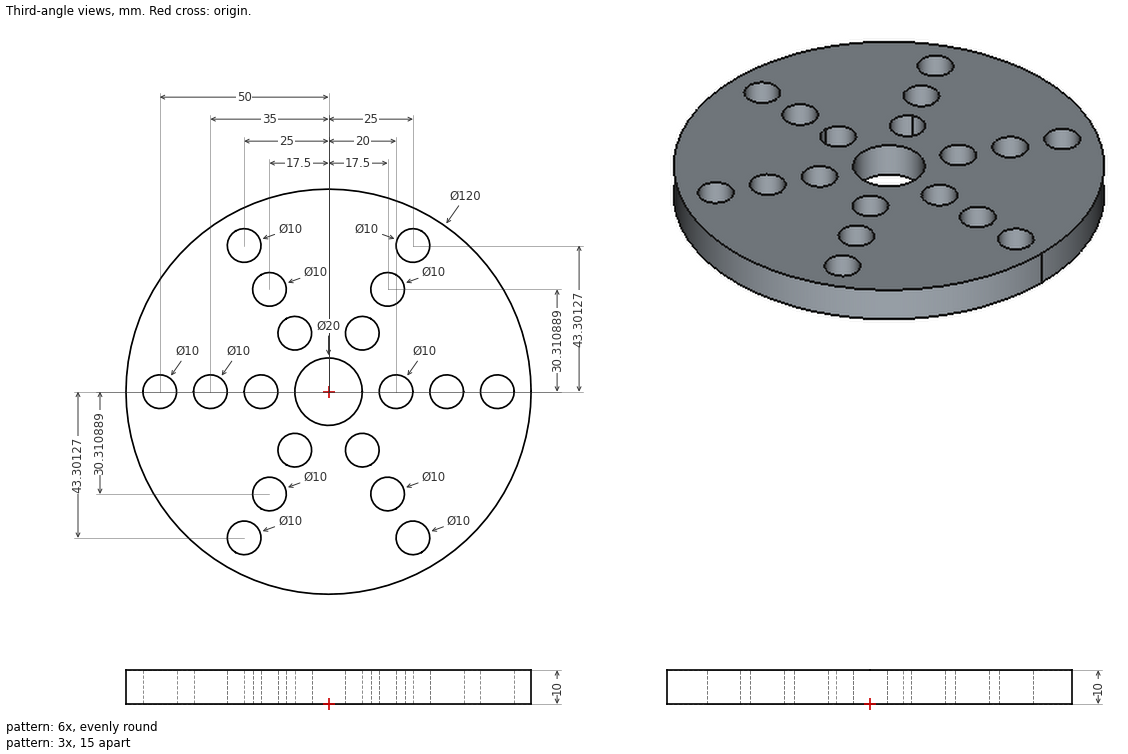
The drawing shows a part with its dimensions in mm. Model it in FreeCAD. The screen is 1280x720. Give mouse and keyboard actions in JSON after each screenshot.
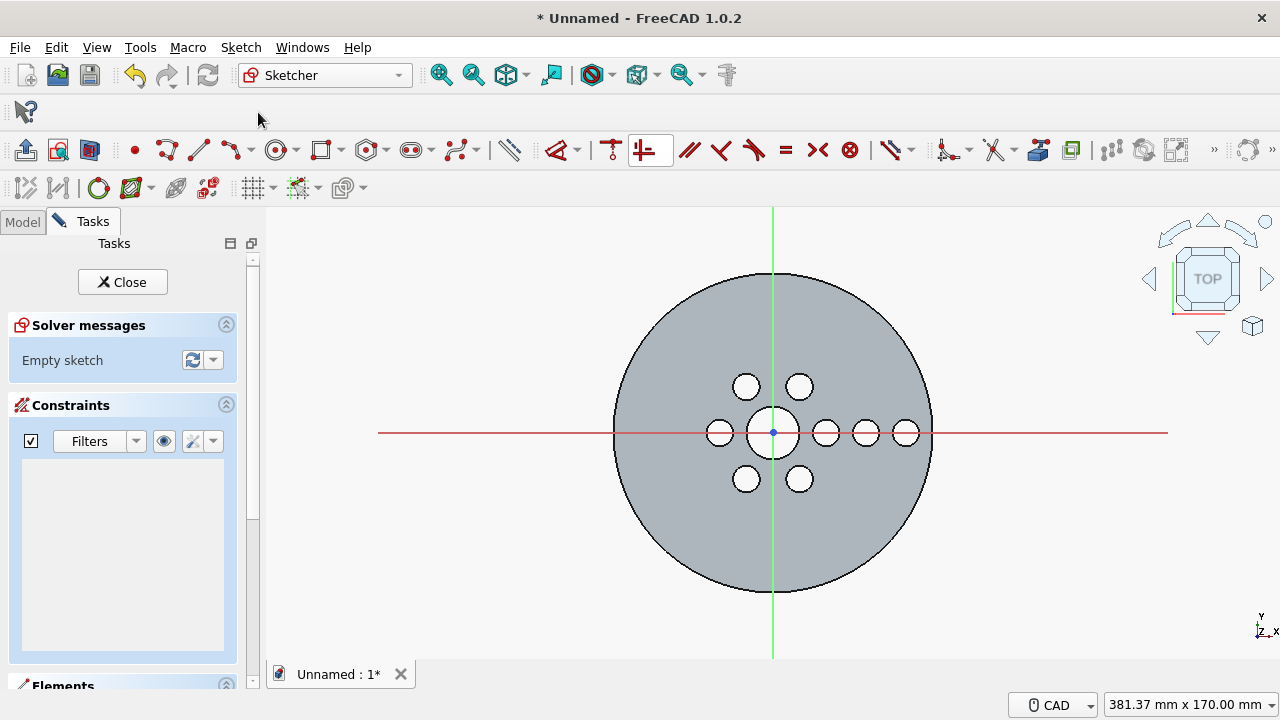
{"action": "scroll", "coordinate": [831, 344], "scroll_direction": "up", "scroll_amount": 12}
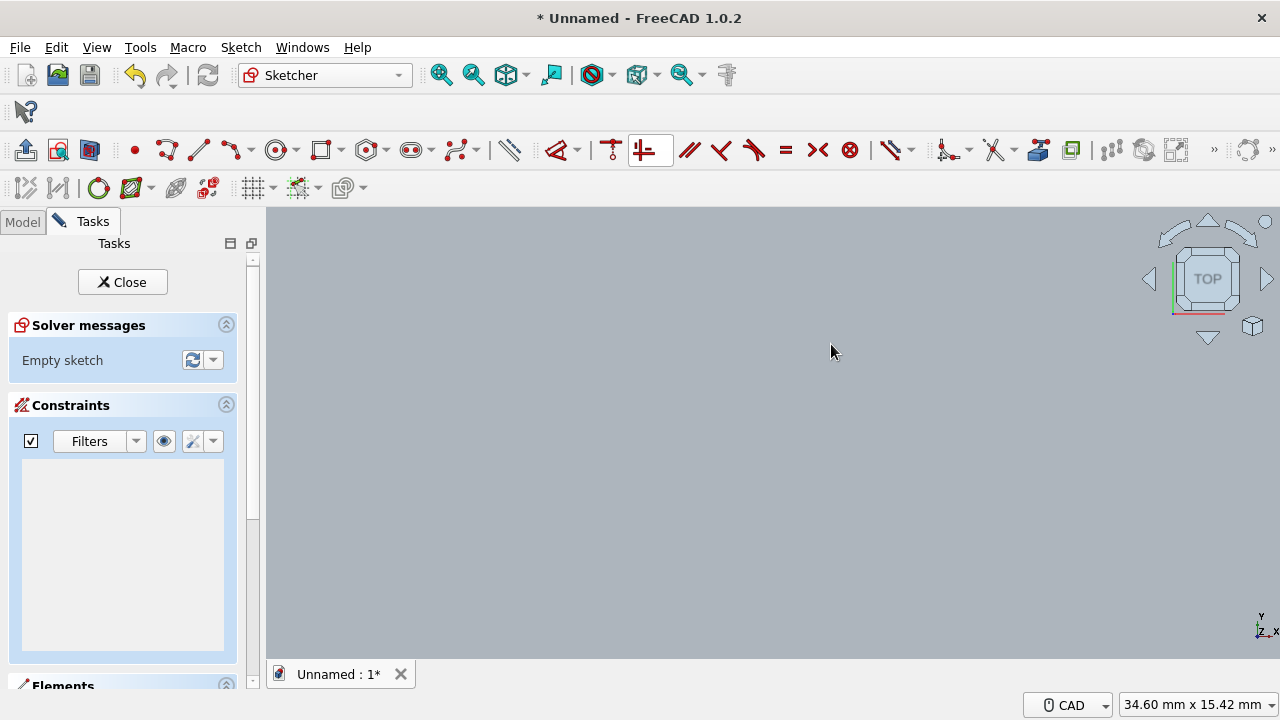
{"action": "left_click", "coordinate": [276, 150]}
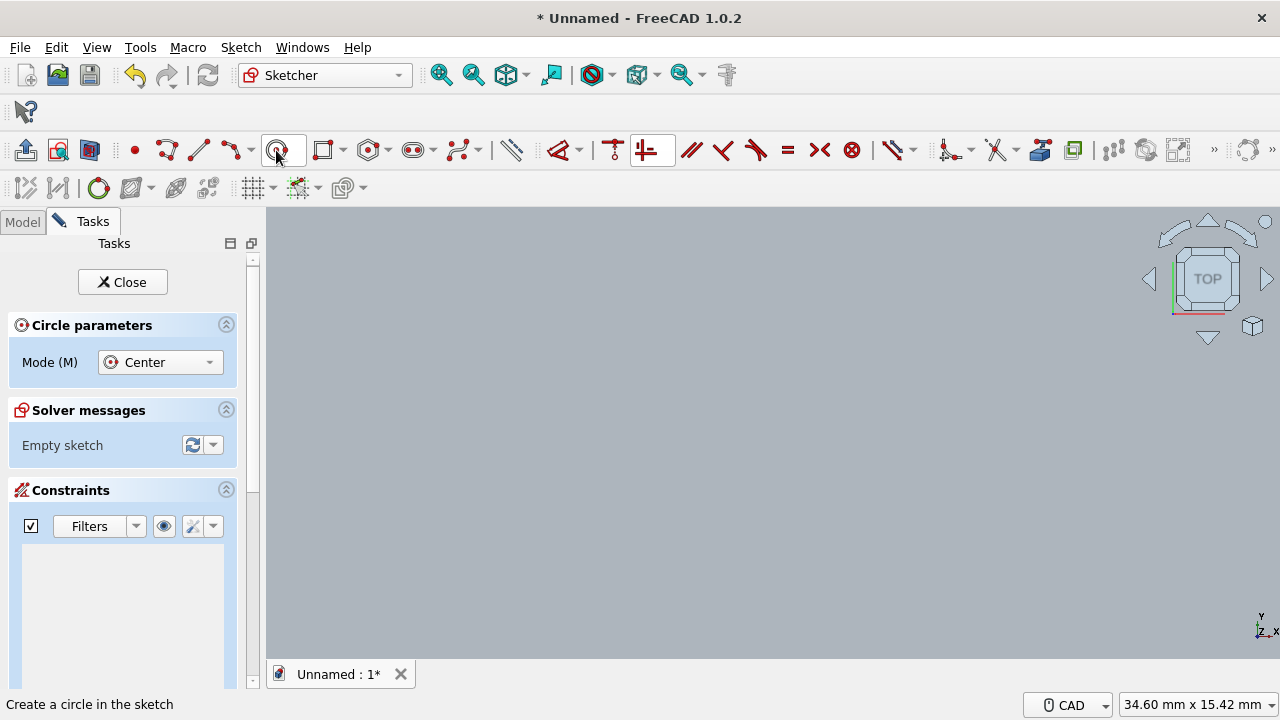
{"action": "left_click", "coordinate": [699, 434]}
{"action": "left_click", "coordinate": [803, 330]}
{"action": "key", "text": "Escape"}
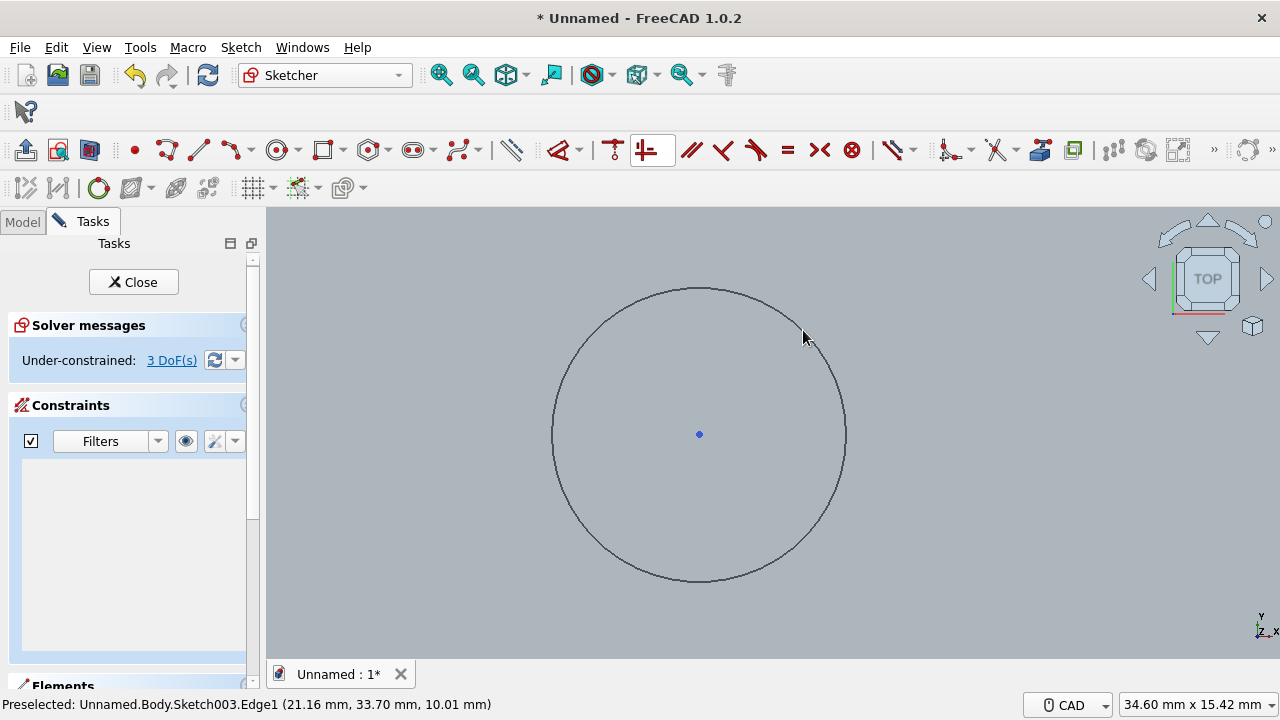
{"action": "left_click", "coordinate": [558, 150]}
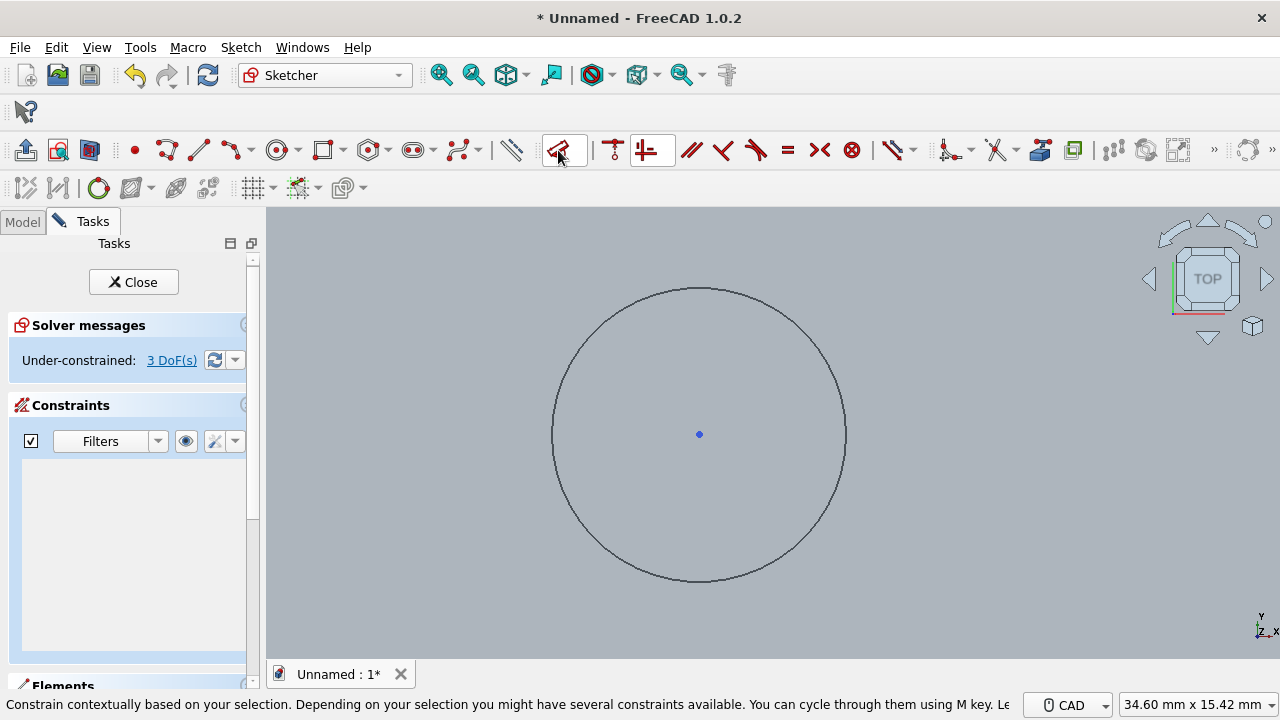
{"action": "left_click", "coordinate": [803, 331]}
{"action": "left_click", "coordinate": [826, 308]}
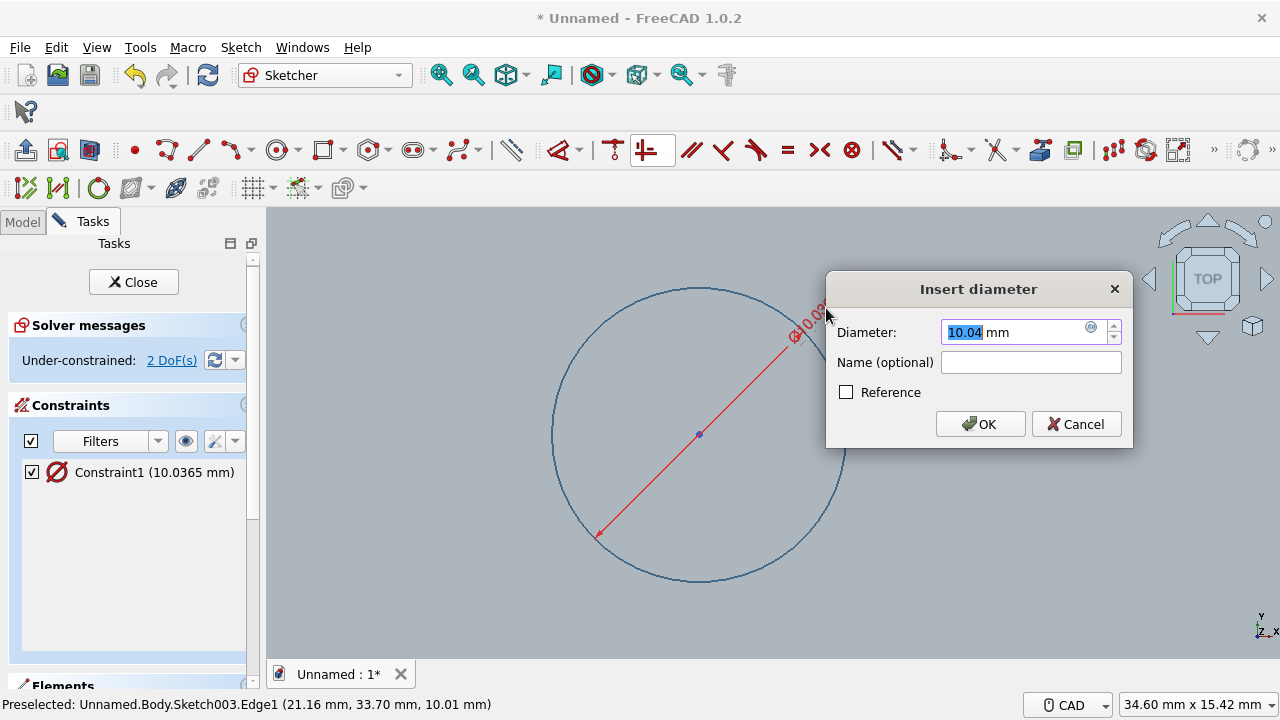
{"action": "type", "text": "10"}
{"action": "key", "text": "Return"}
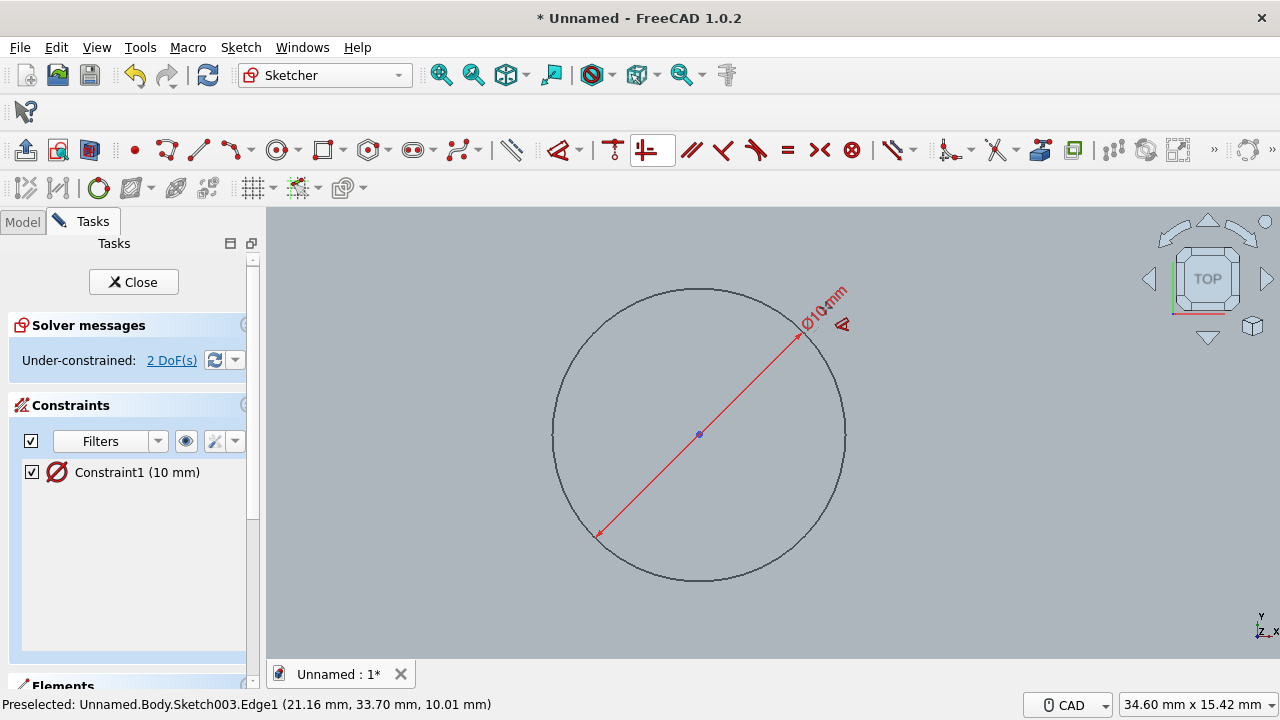
{"action": "left_click", "coordinate": [699, 435]}
{"action": "left_click", "coordinate": [496, 401]}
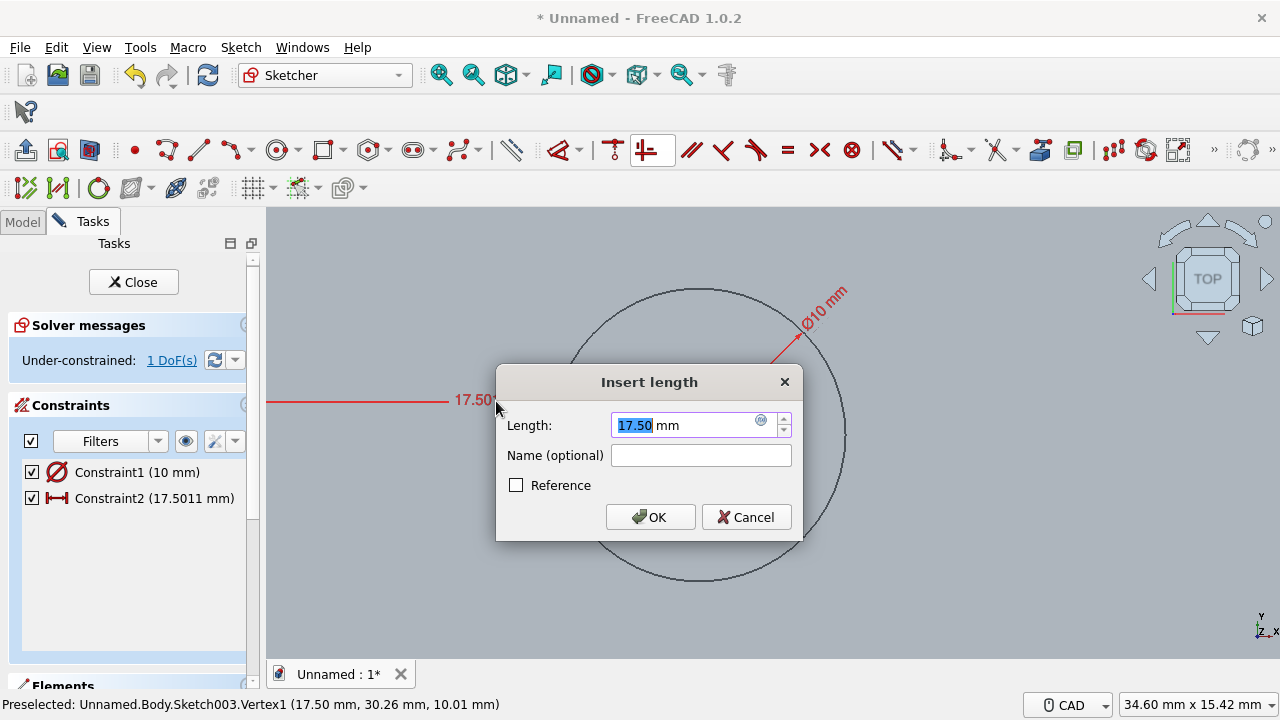
{"action": "type", "text": "17.5"}
{"action": "key", "text": "Return"}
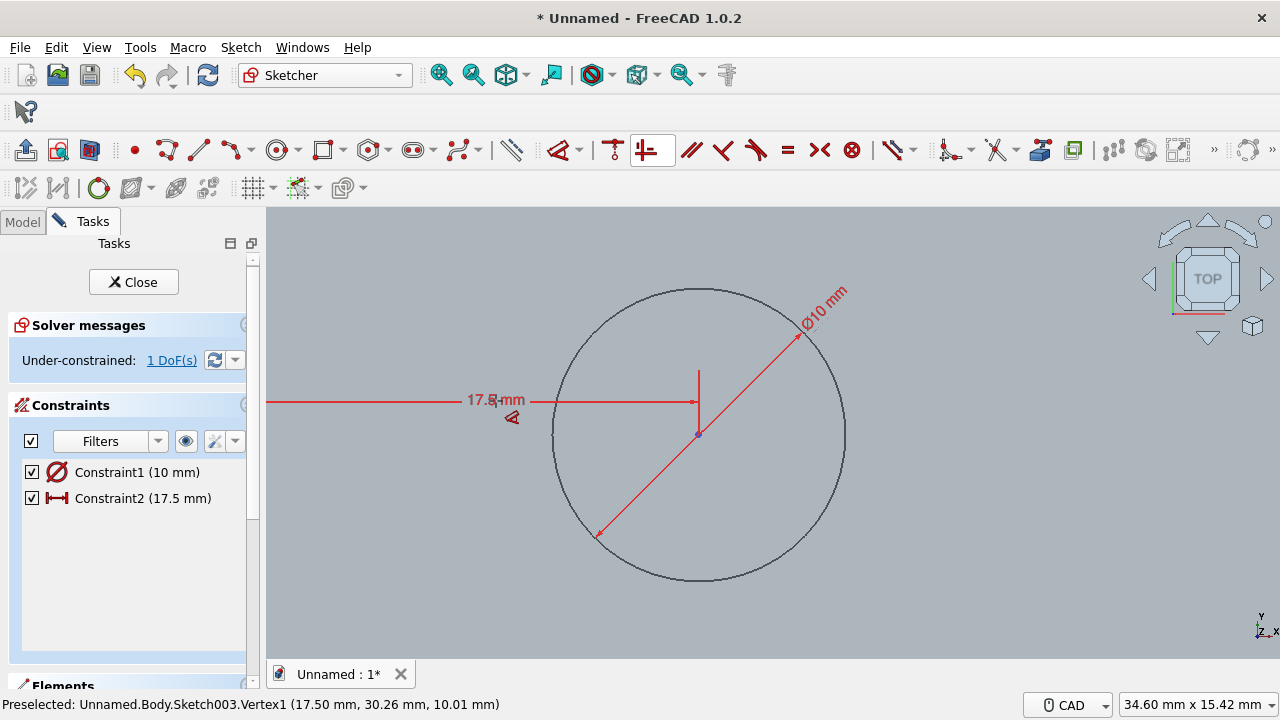
{"action": "left_click", "coordinate": [699, 435]}
{"action": "left_click", "coordinate": [733, 533]}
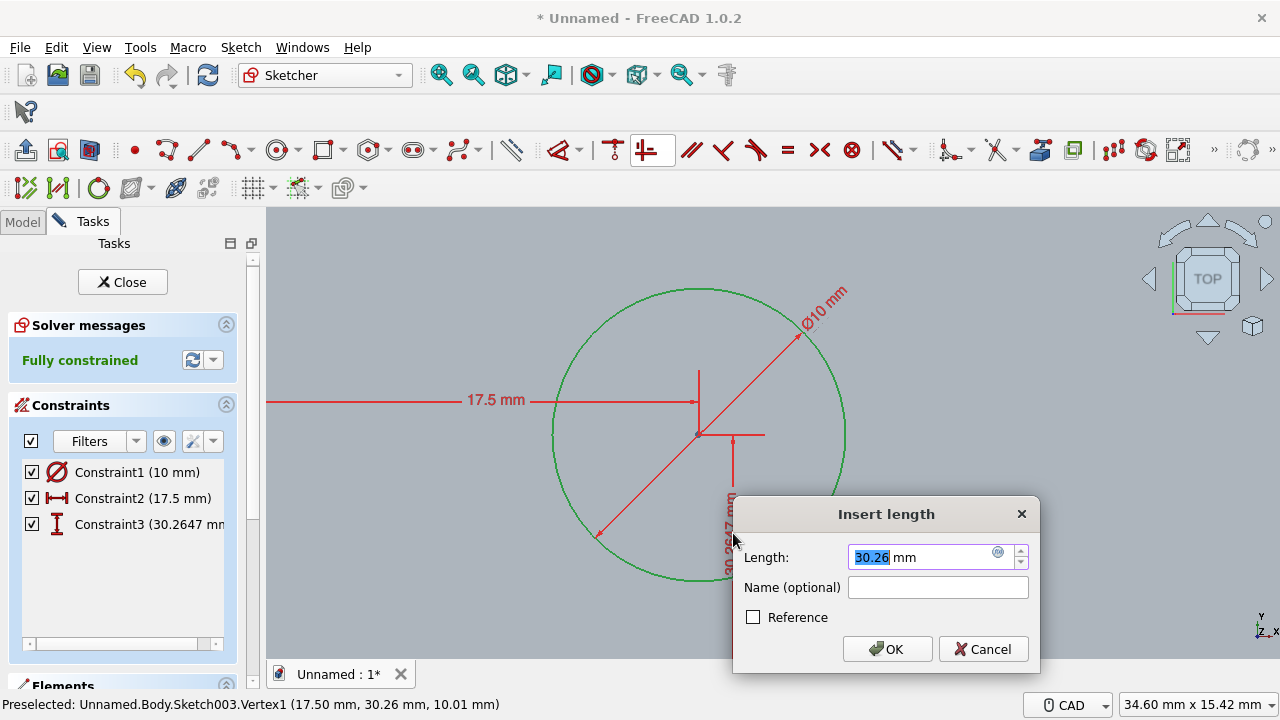
{"action": "type", "text": "30.310889"}
{"action": "key", "text": "Return"}
{"action": "key", "text": "Escape"}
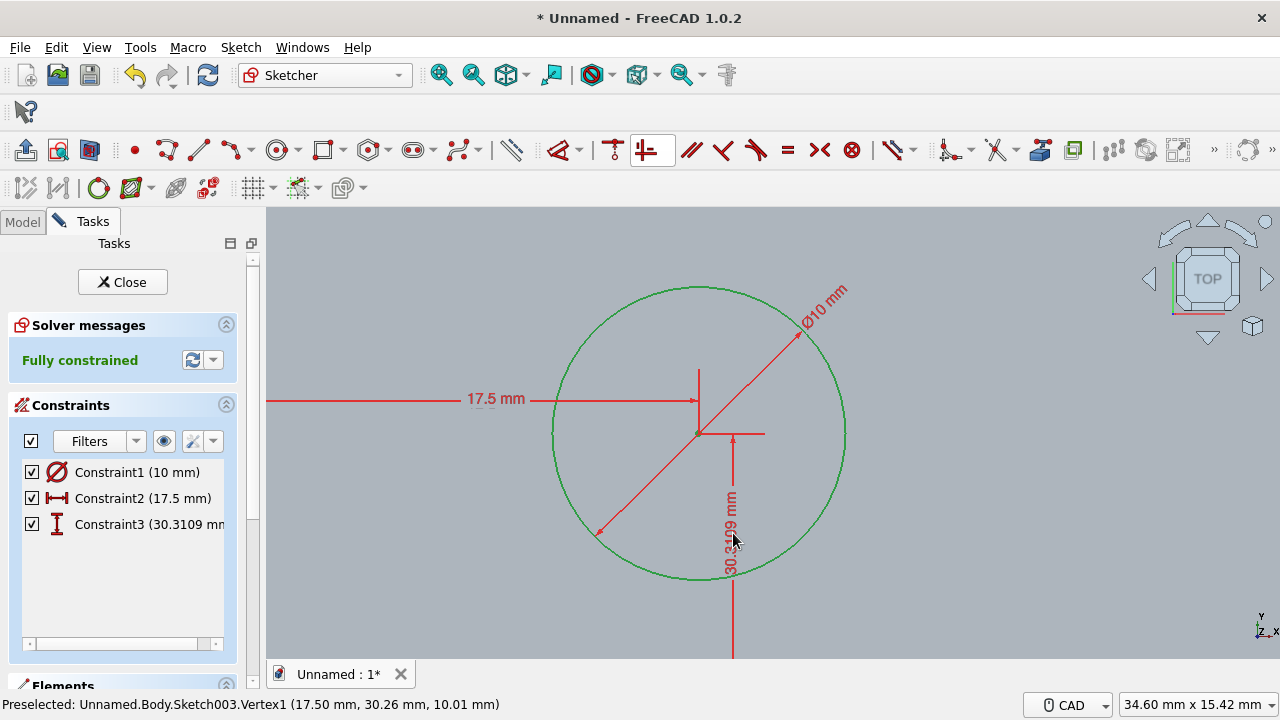
{"action": "left_click", "coordinate": [123, 282]}